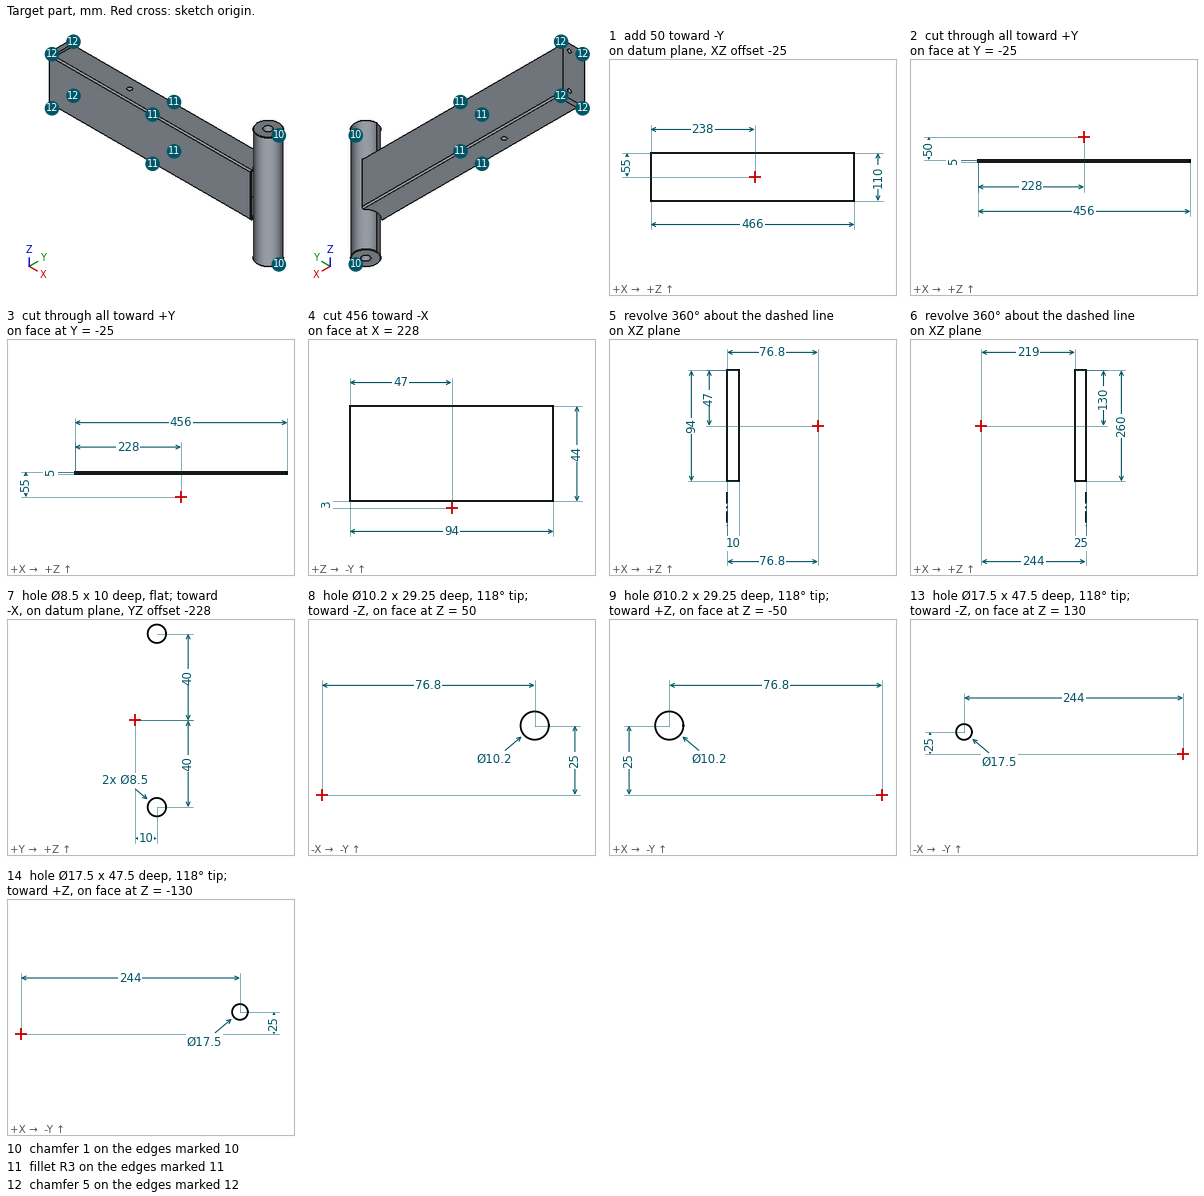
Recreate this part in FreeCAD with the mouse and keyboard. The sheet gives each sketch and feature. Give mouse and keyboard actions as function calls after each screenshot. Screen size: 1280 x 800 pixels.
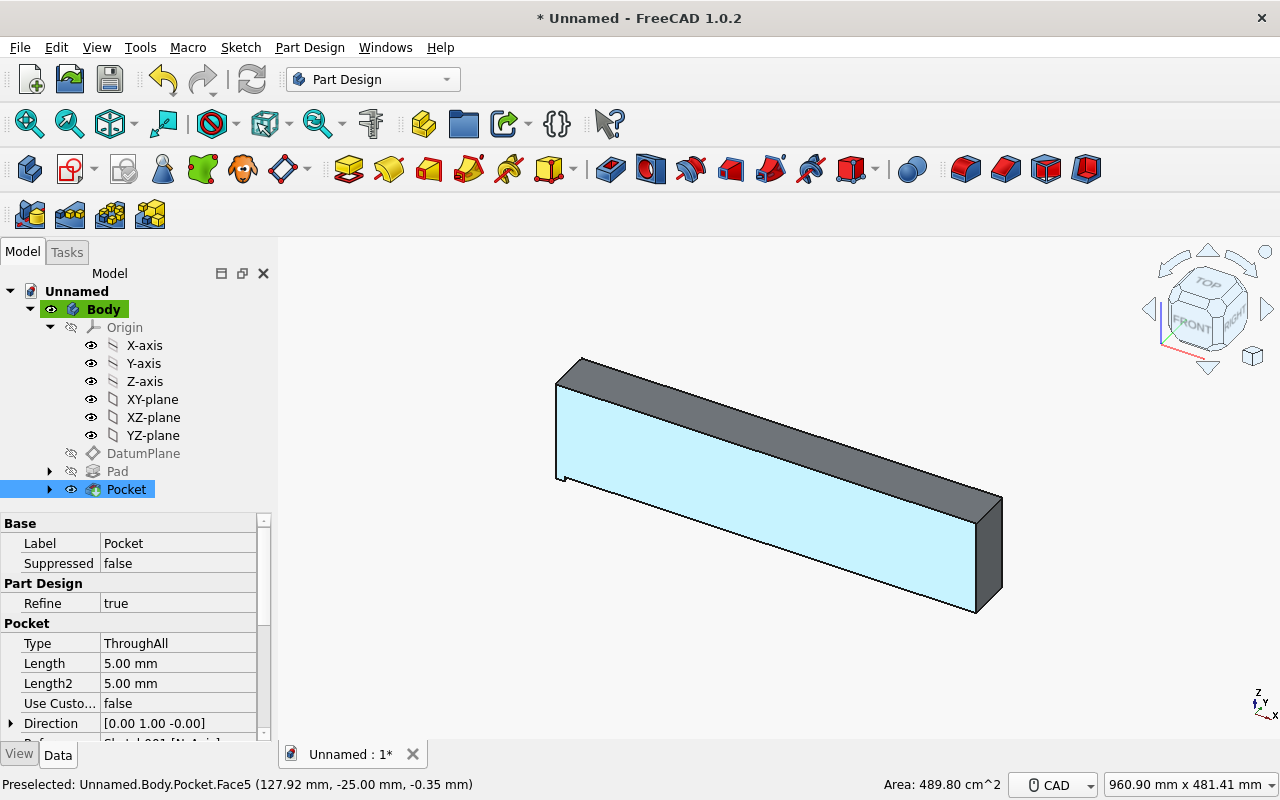
click(70, 170)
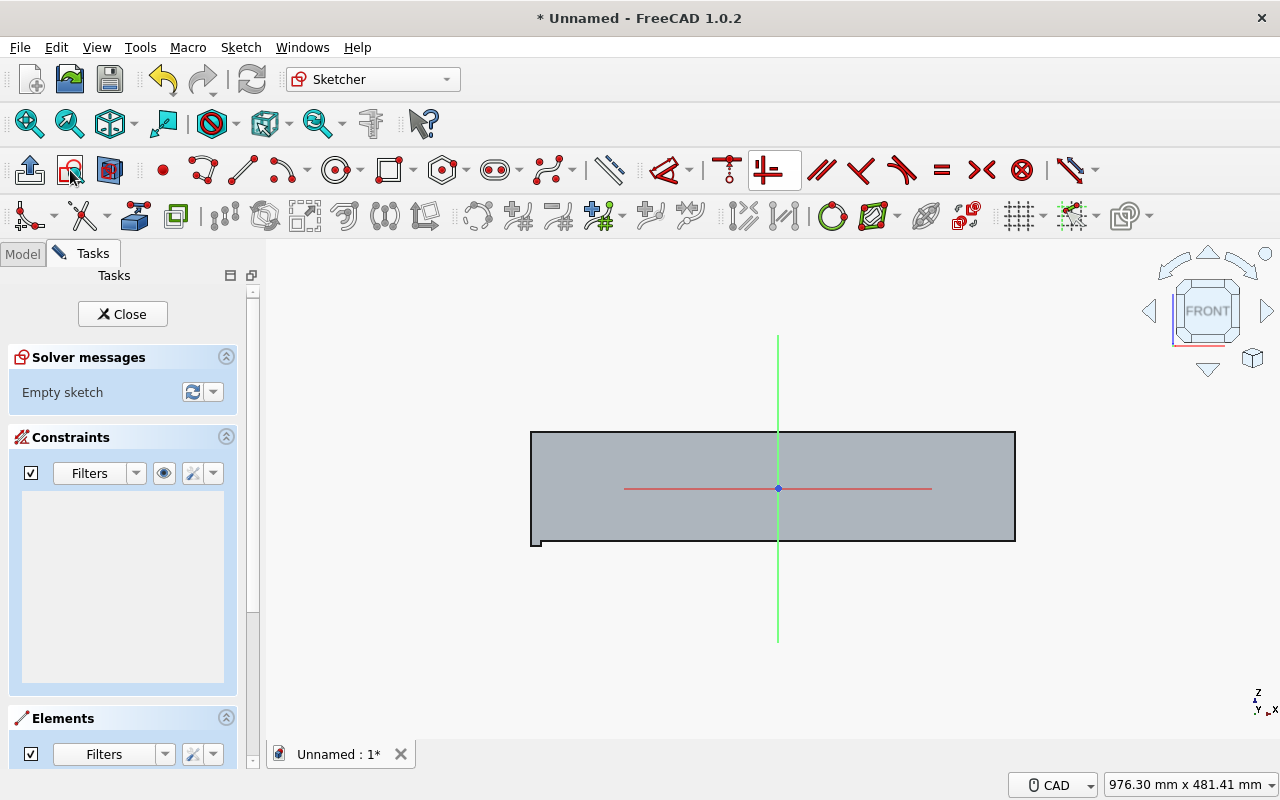
click(390, 170)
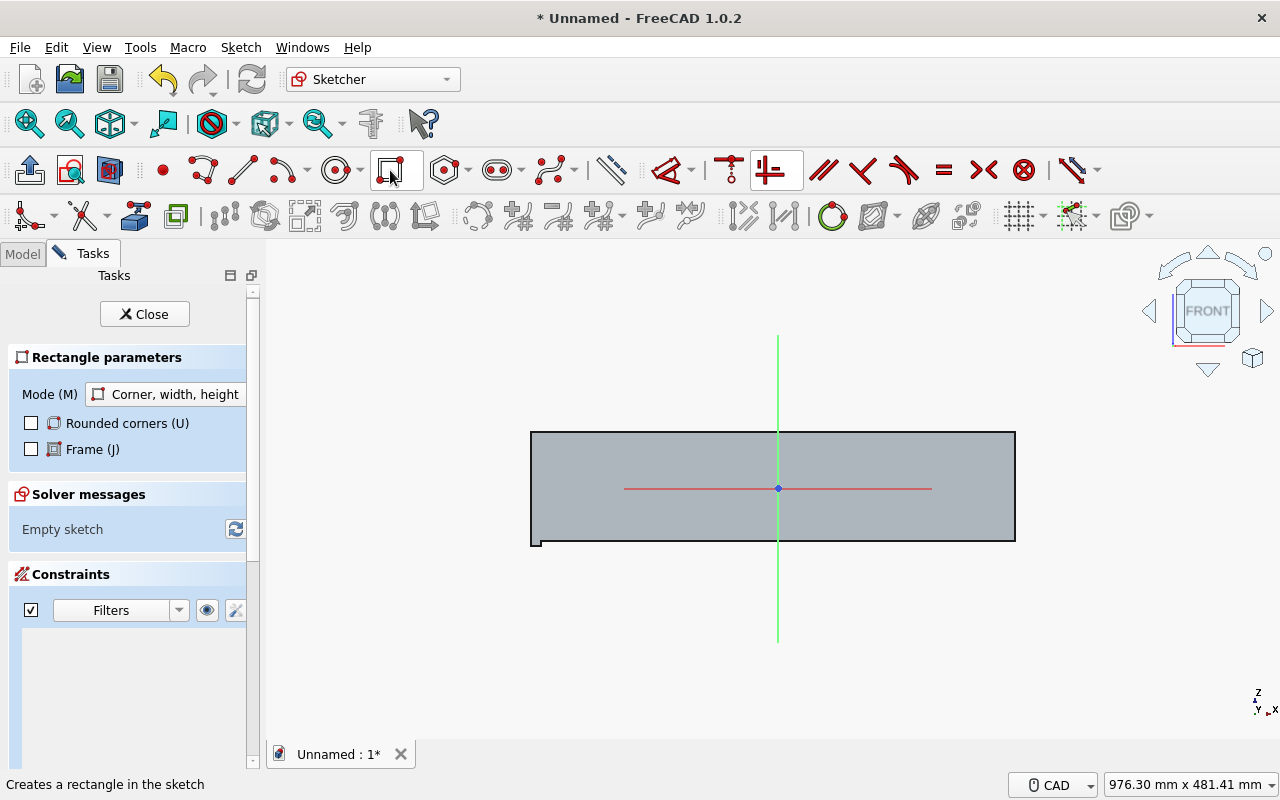
scroll(541, 432, up, 6)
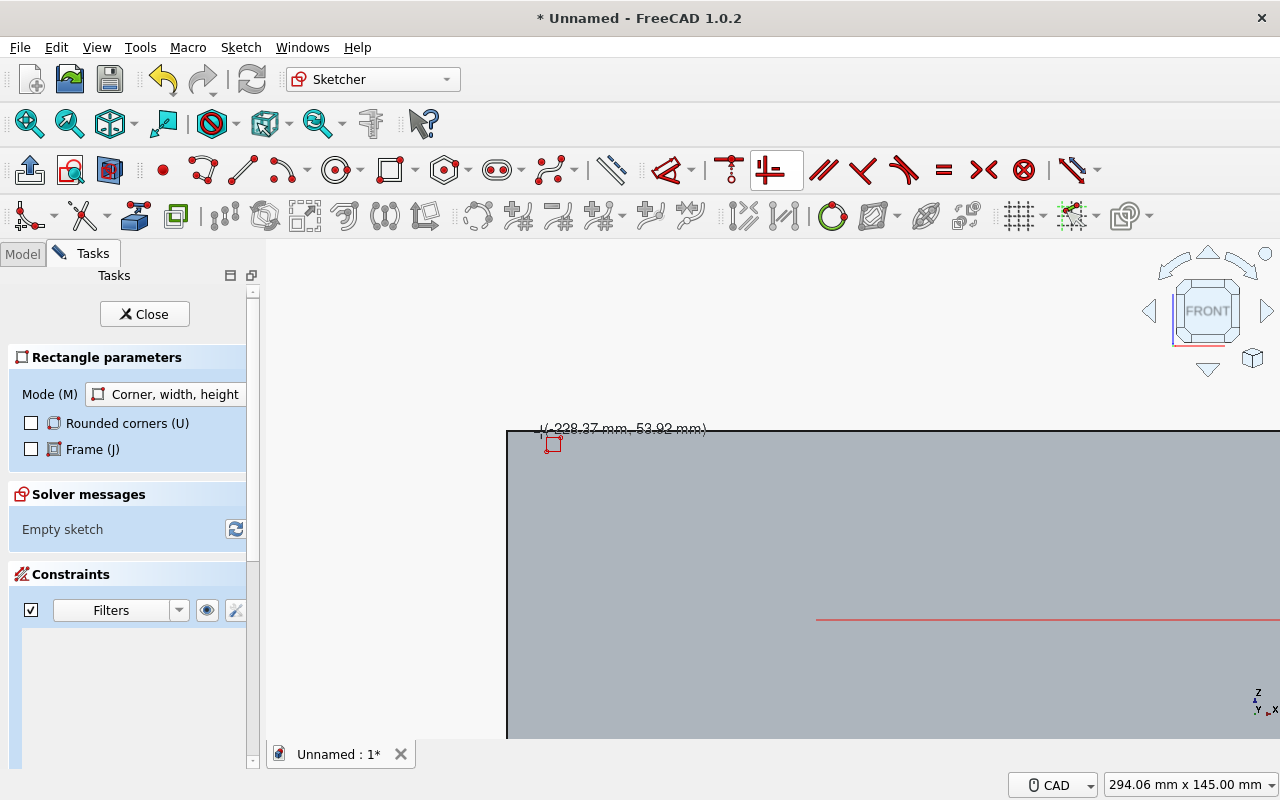
click(542, 431)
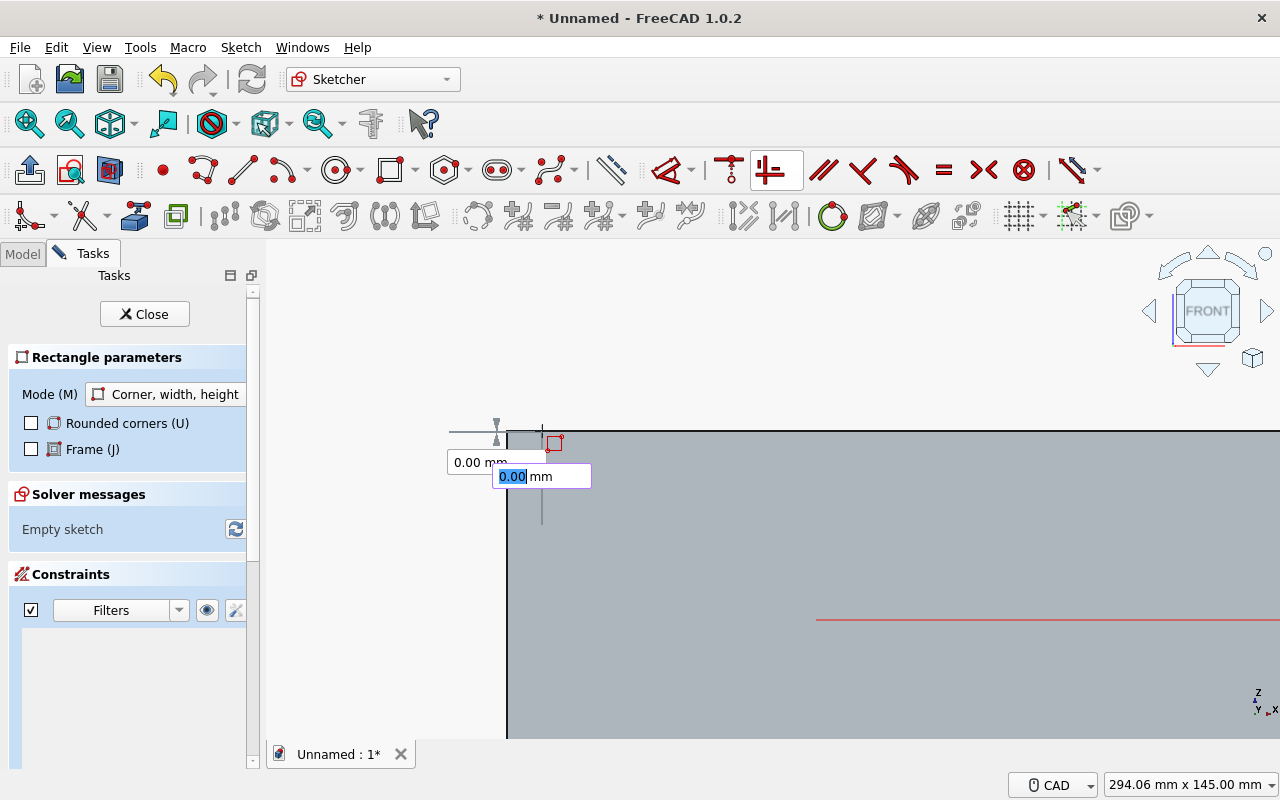
scroll(342, 468, down, 5)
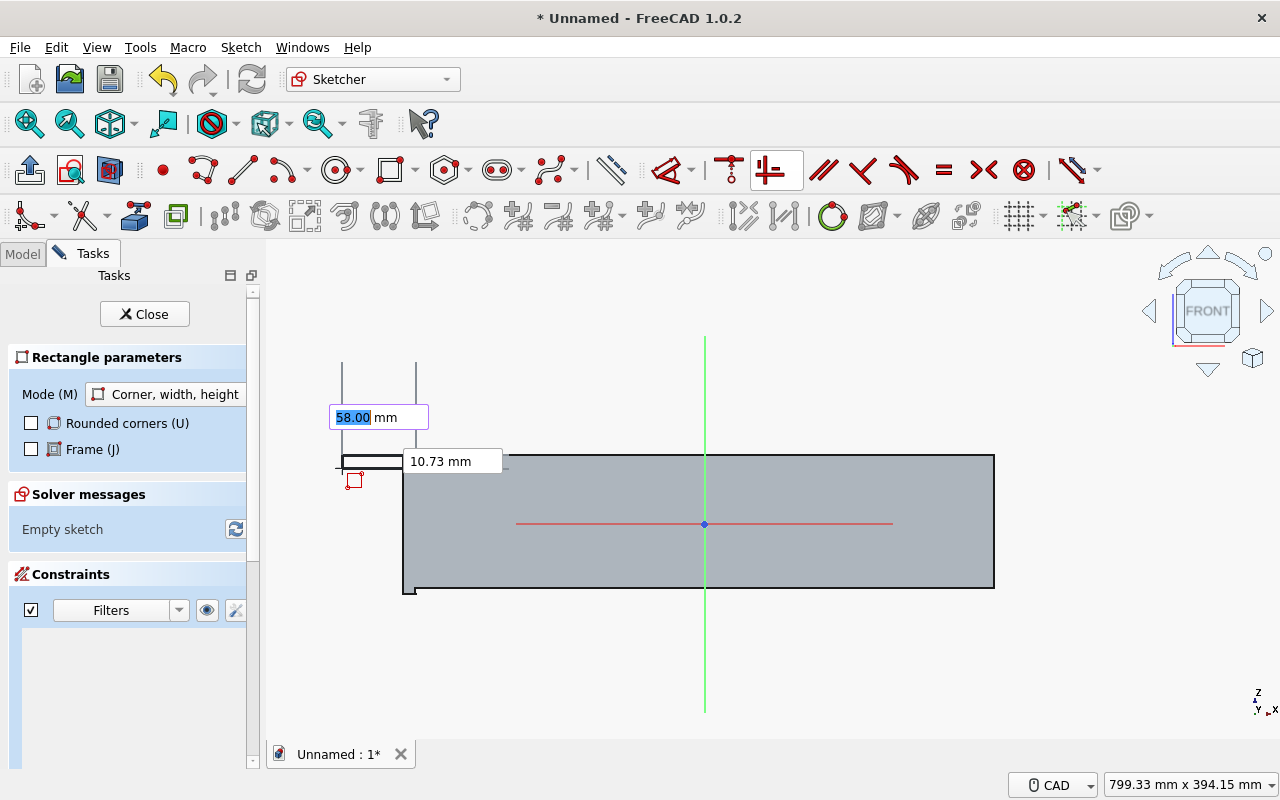
click(994, 461)
key(Escape)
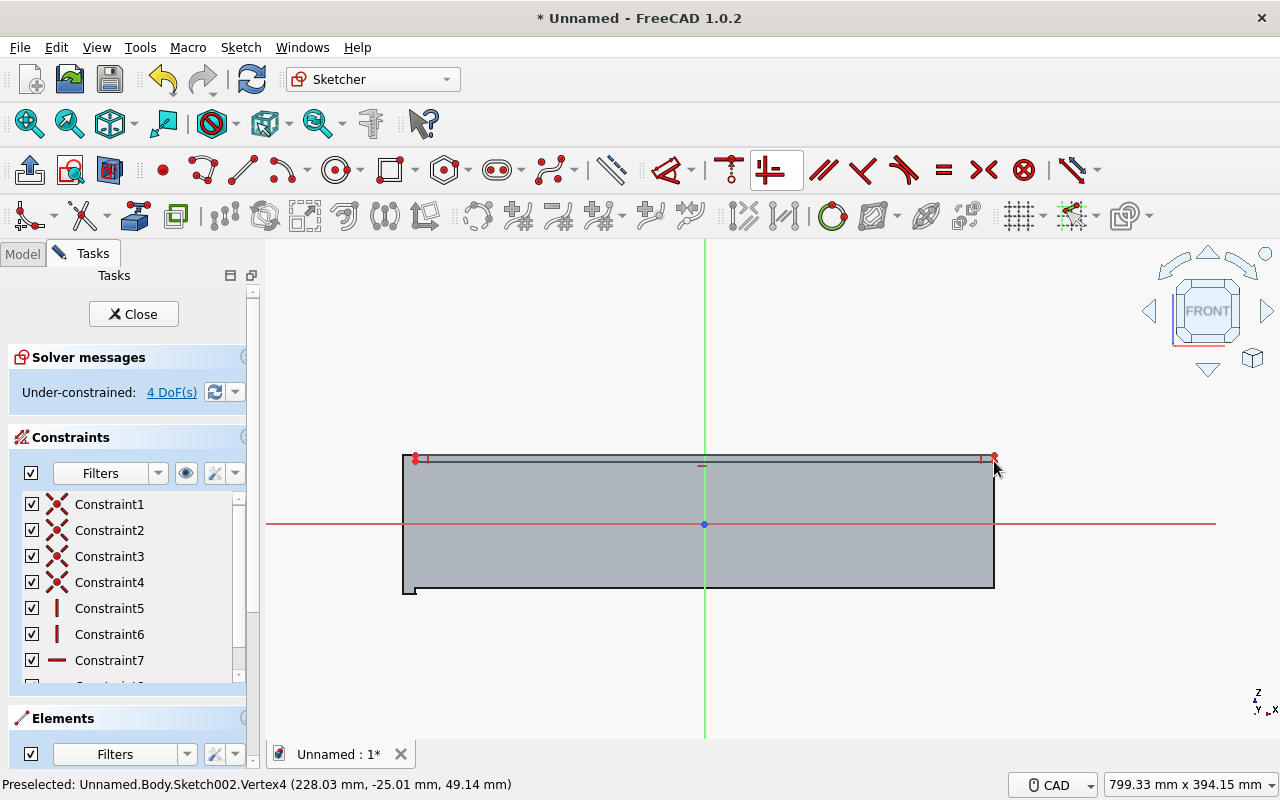
click(666, 170)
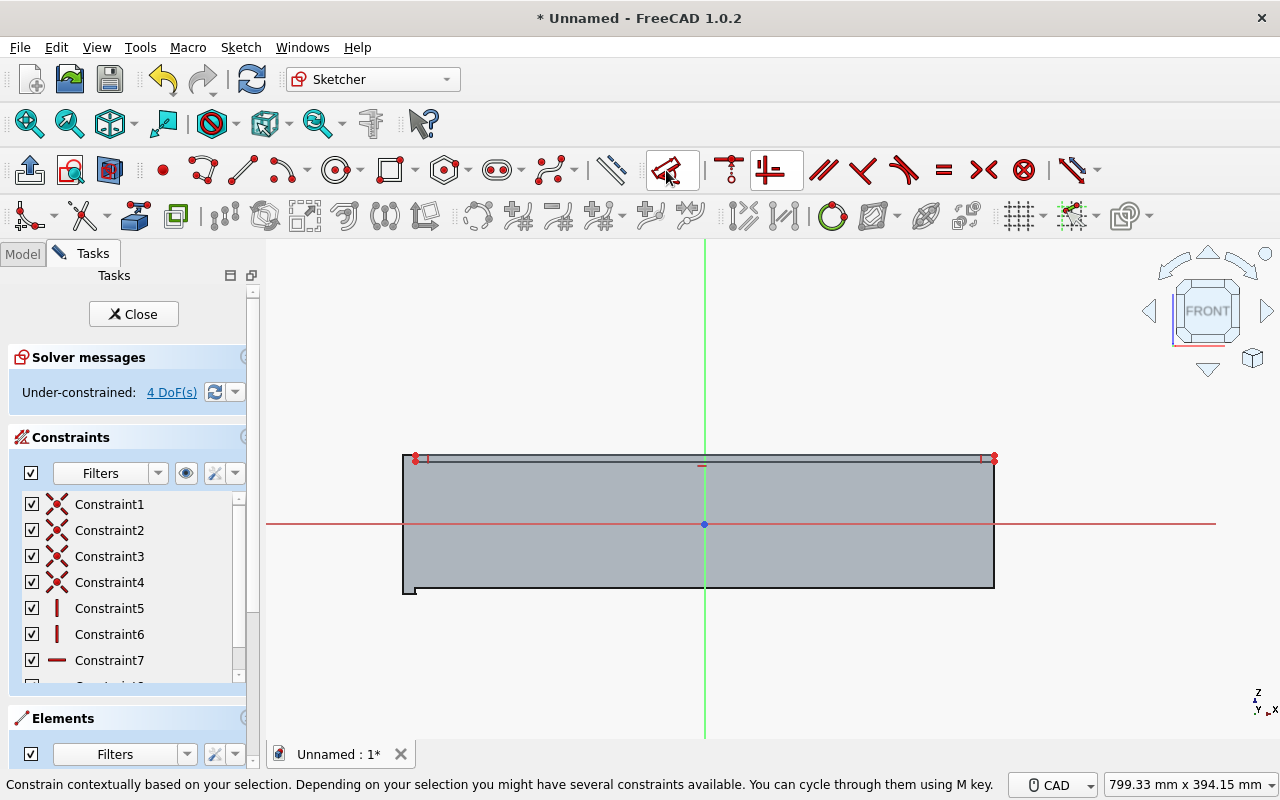
scroll(416, 459, up, 10)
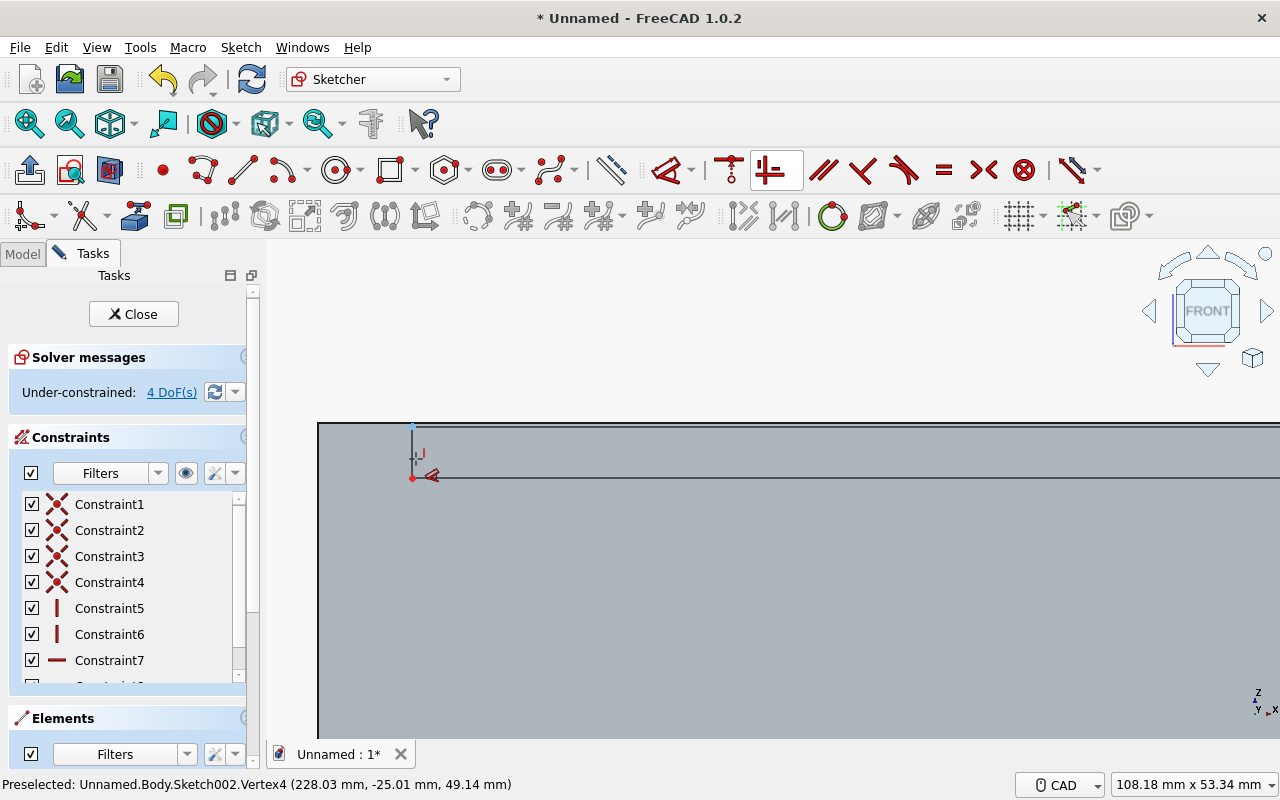
click(412, 453)
click(378, 453)